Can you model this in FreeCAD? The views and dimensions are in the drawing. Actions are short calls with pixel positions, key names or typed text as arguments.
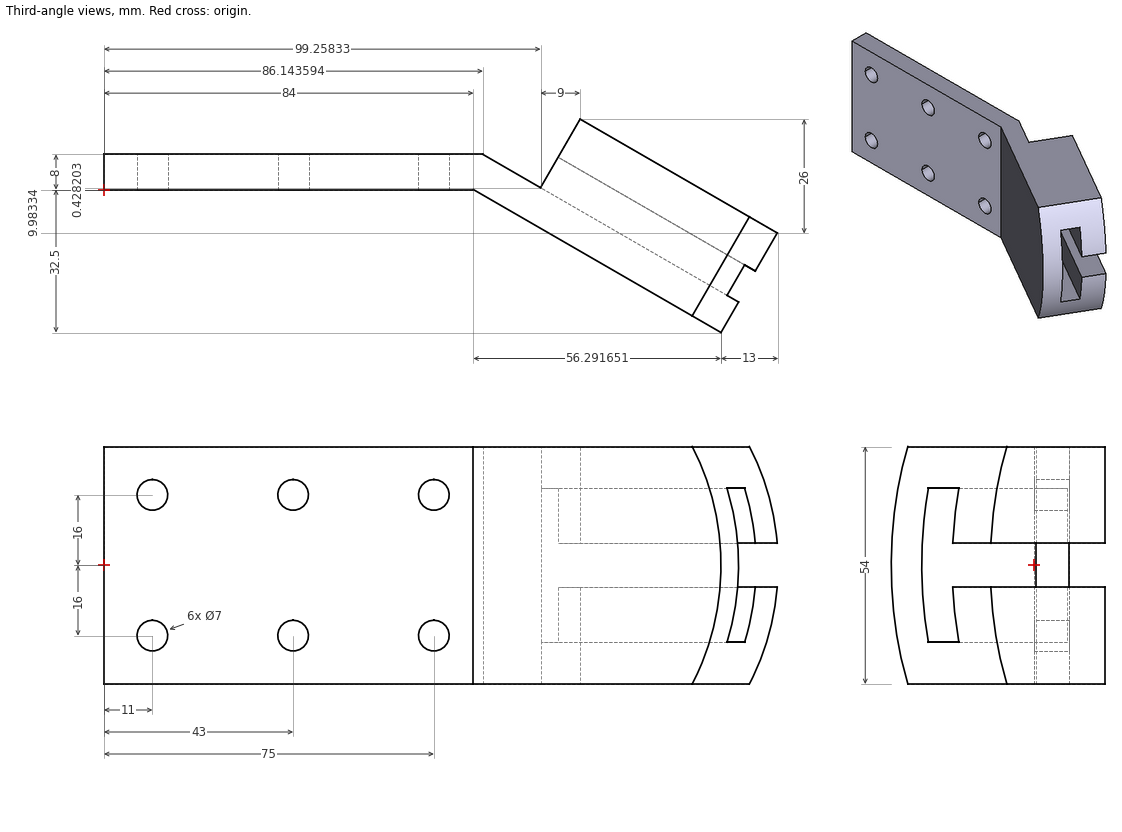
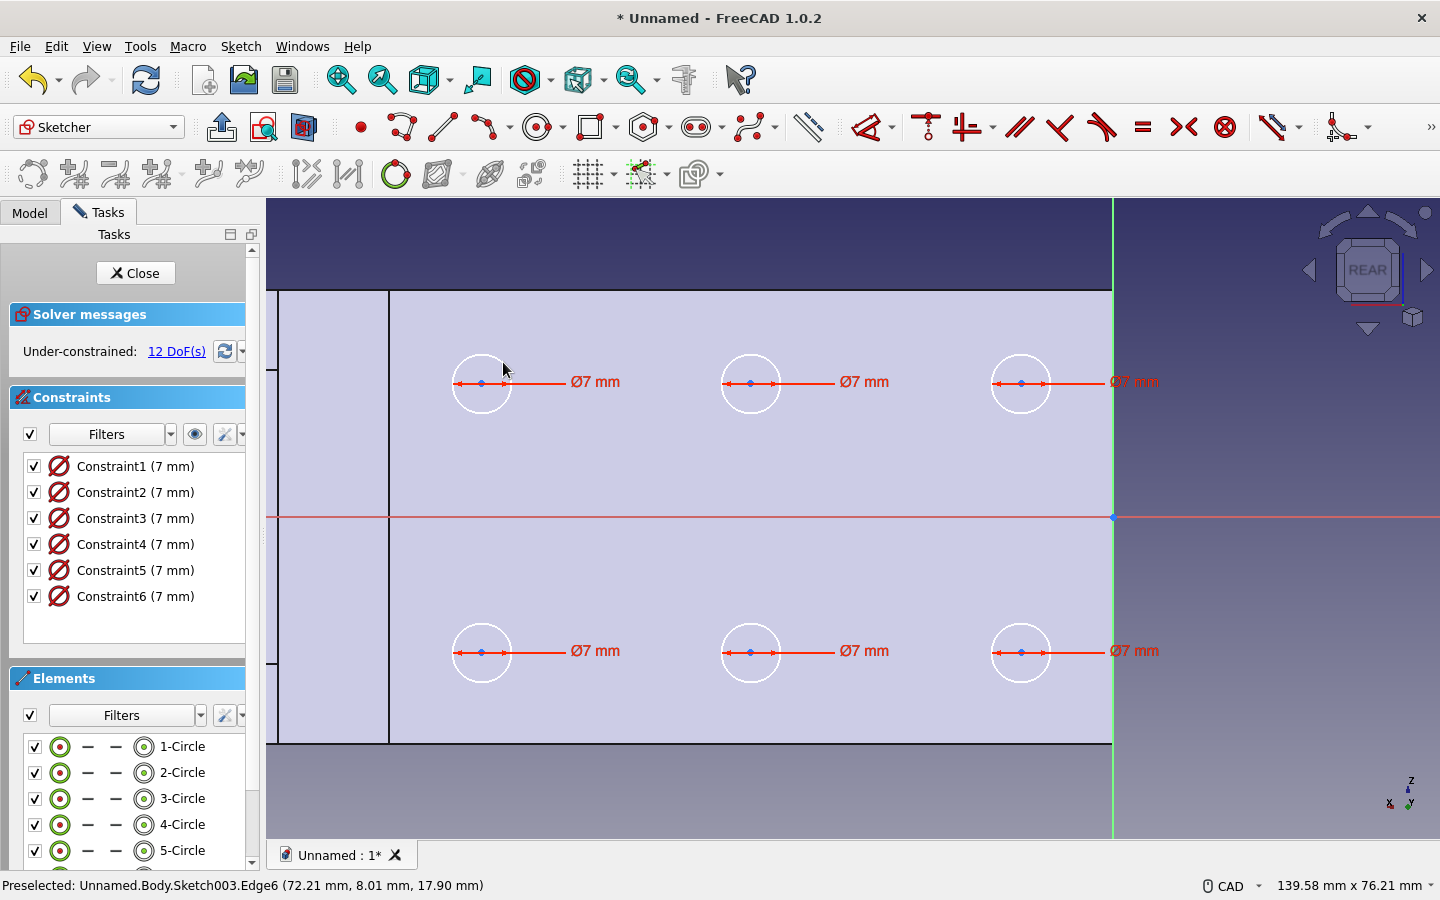
click(1021, 653)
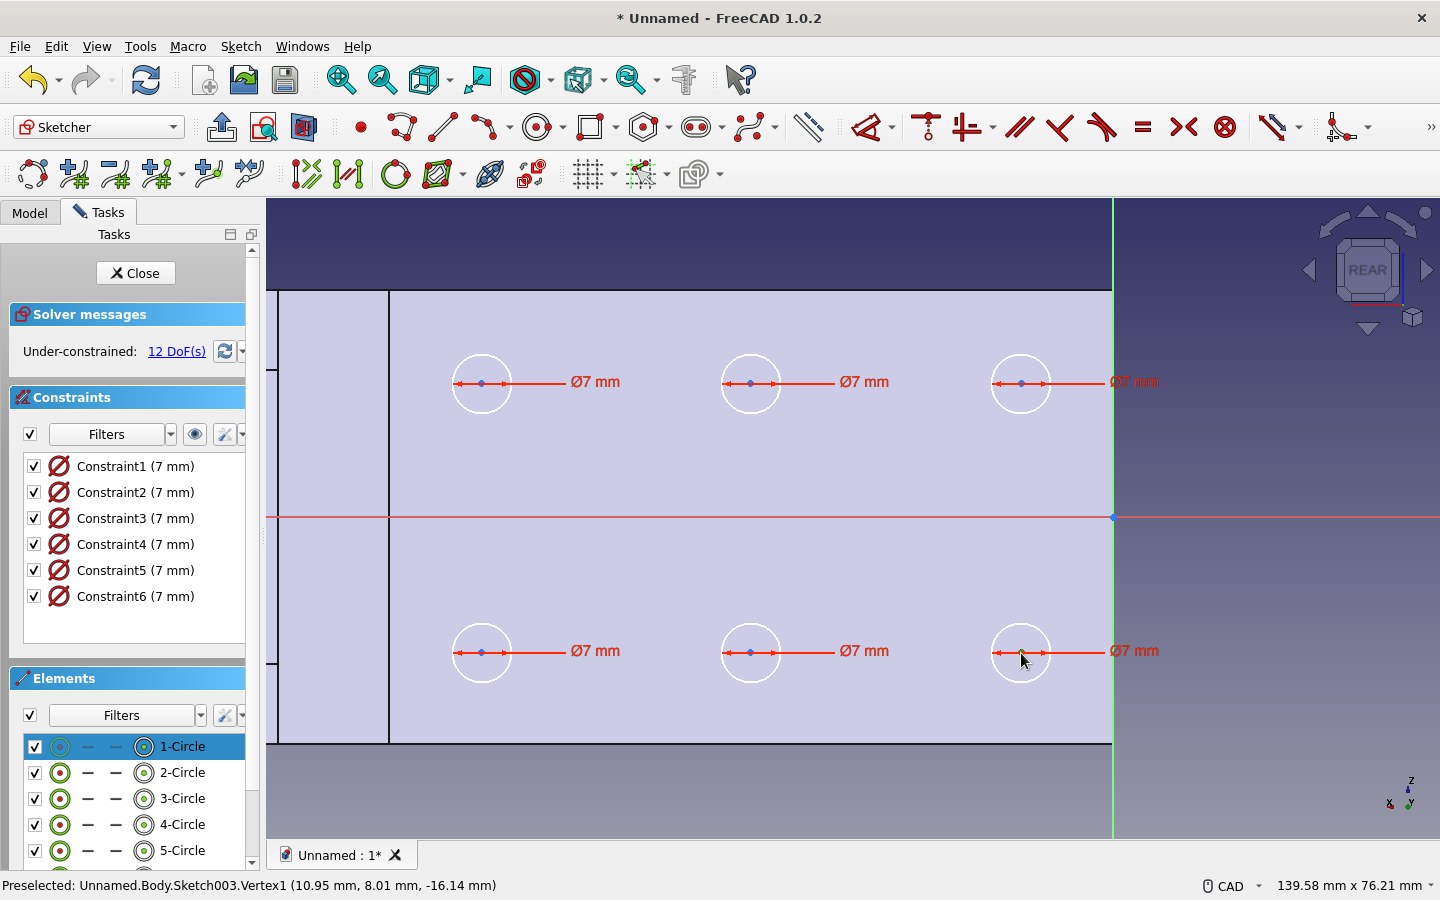
click(751, 653)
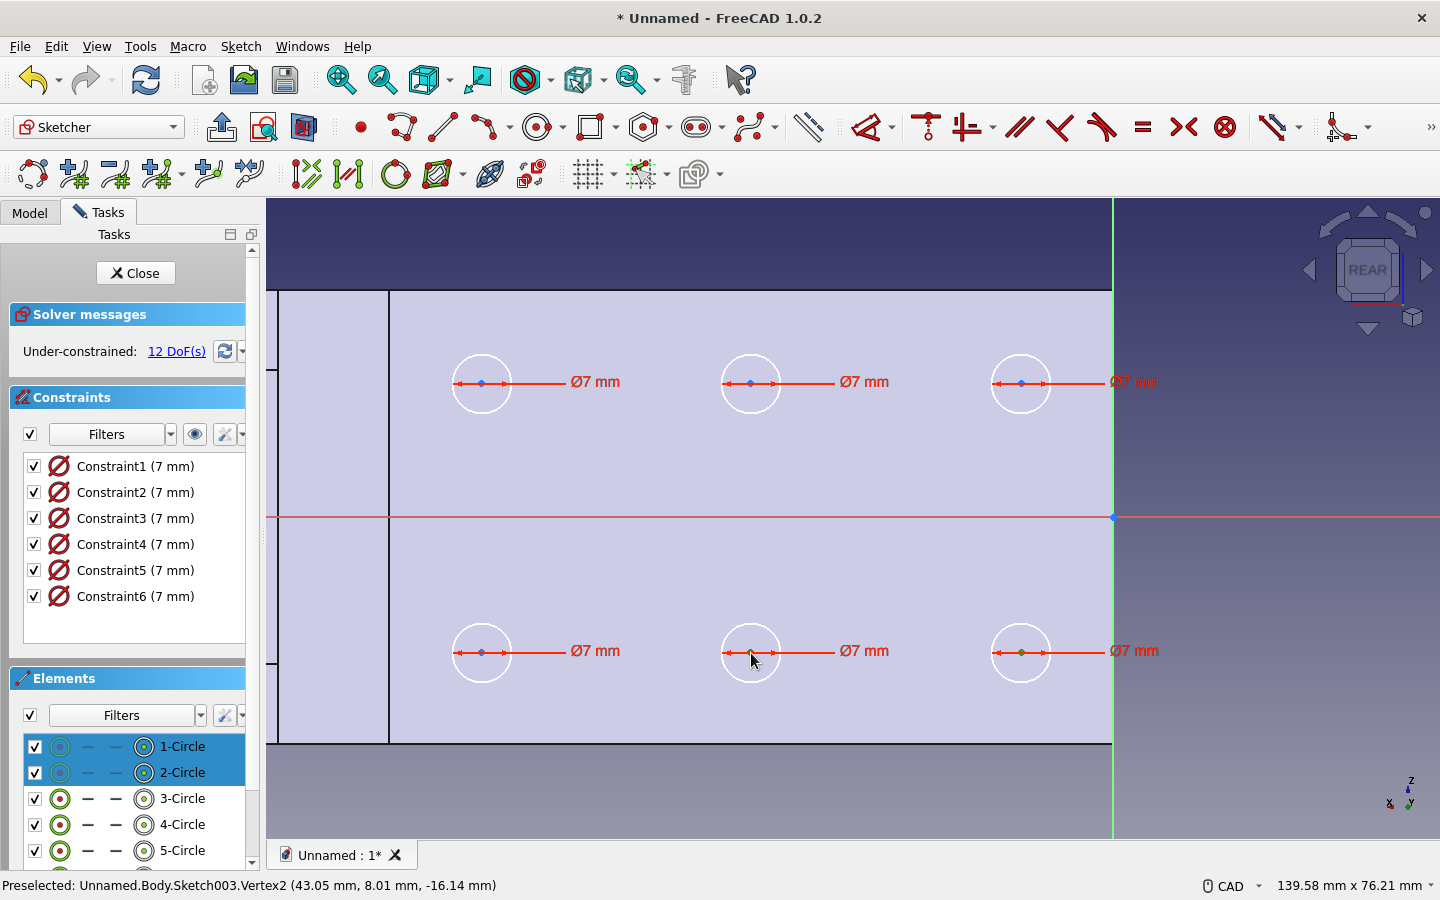
key(h)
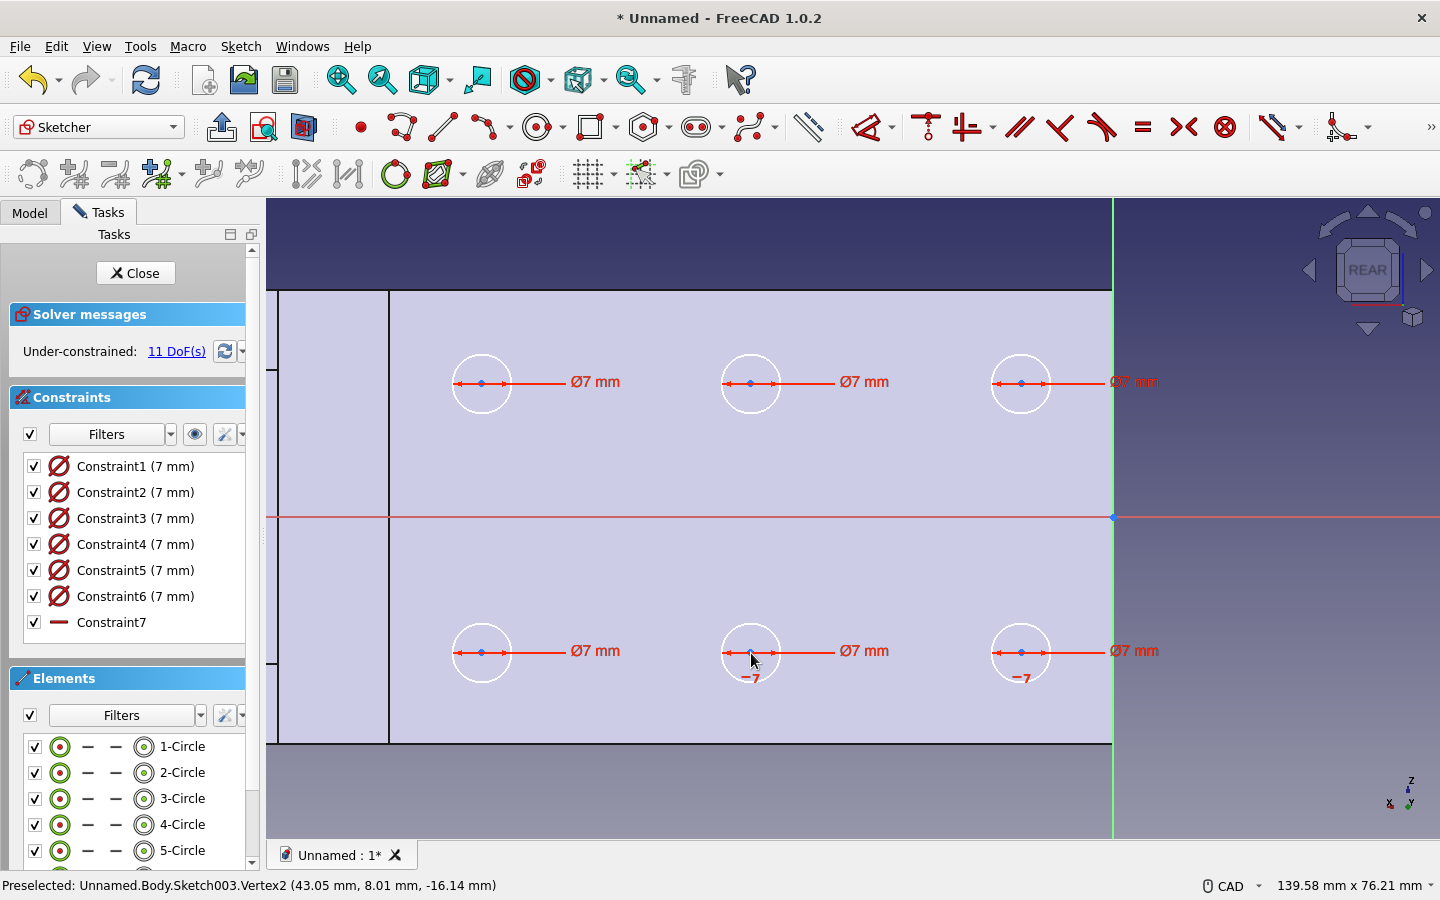
click(751, 653)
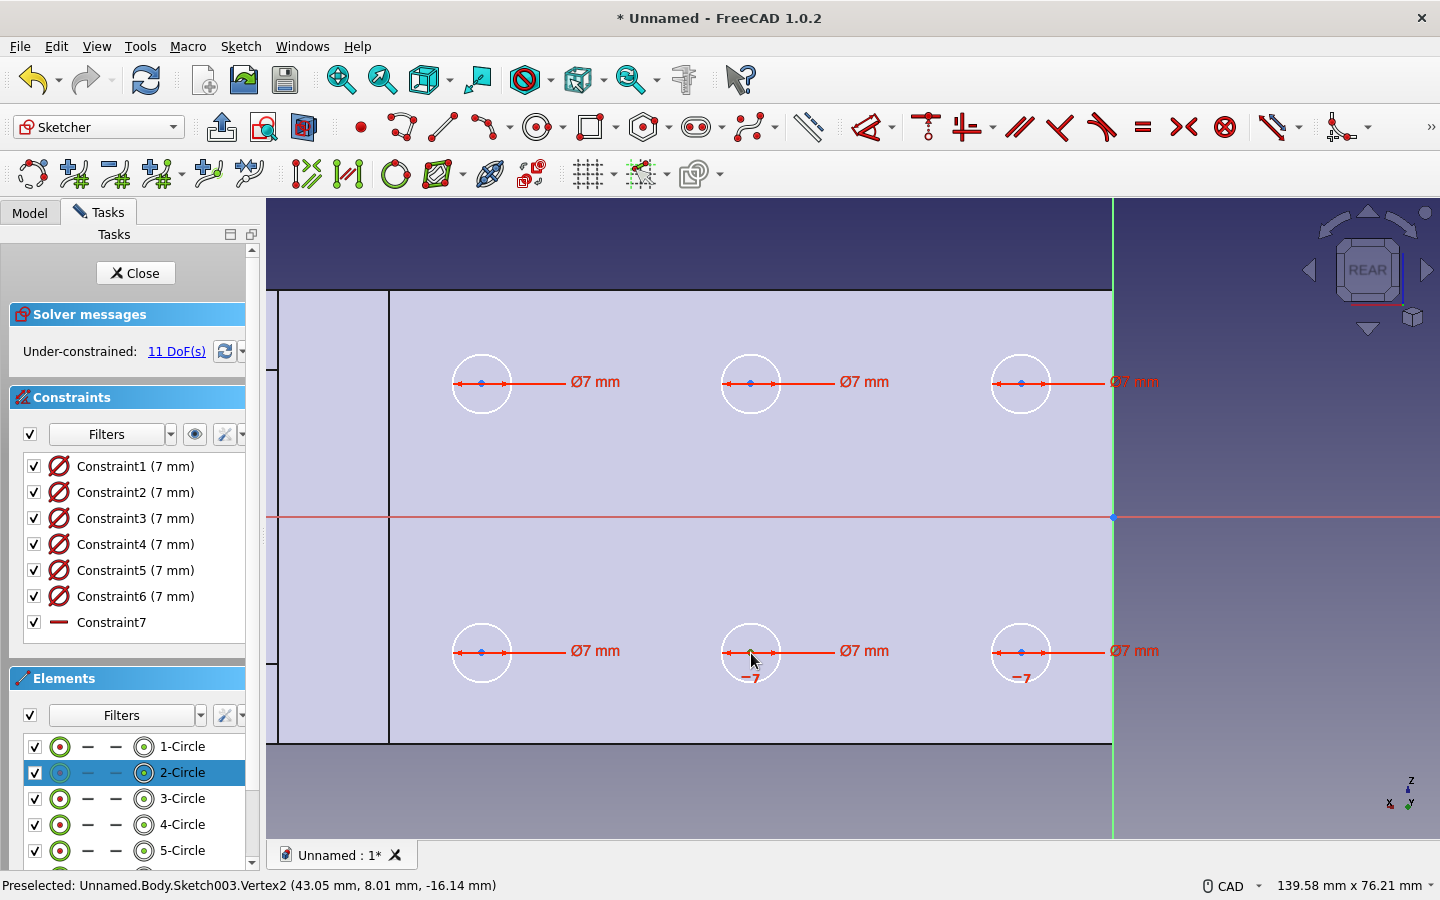
click(482, 653)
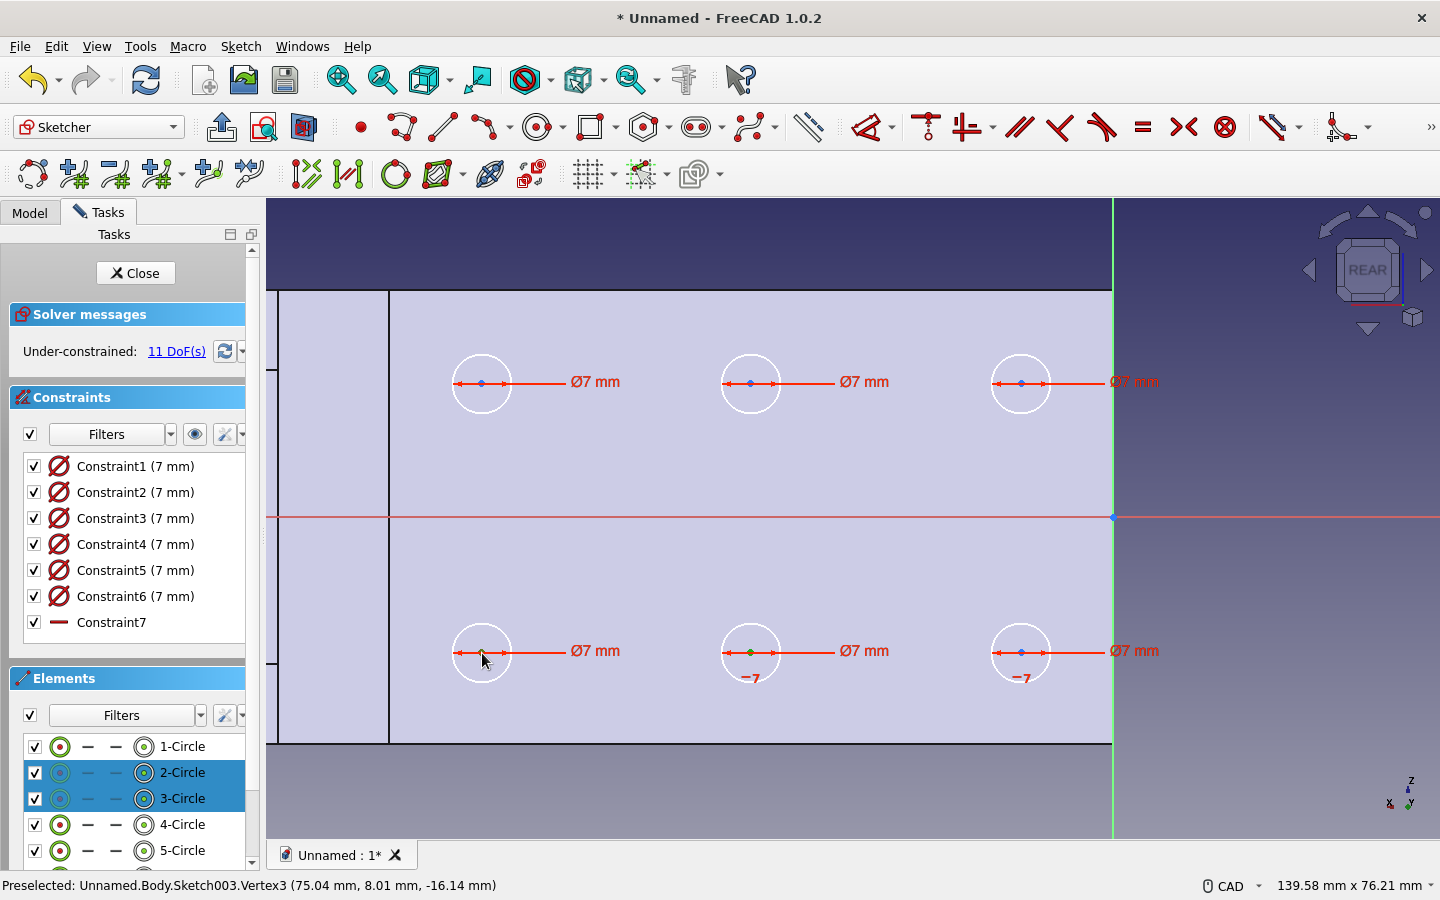
key(h)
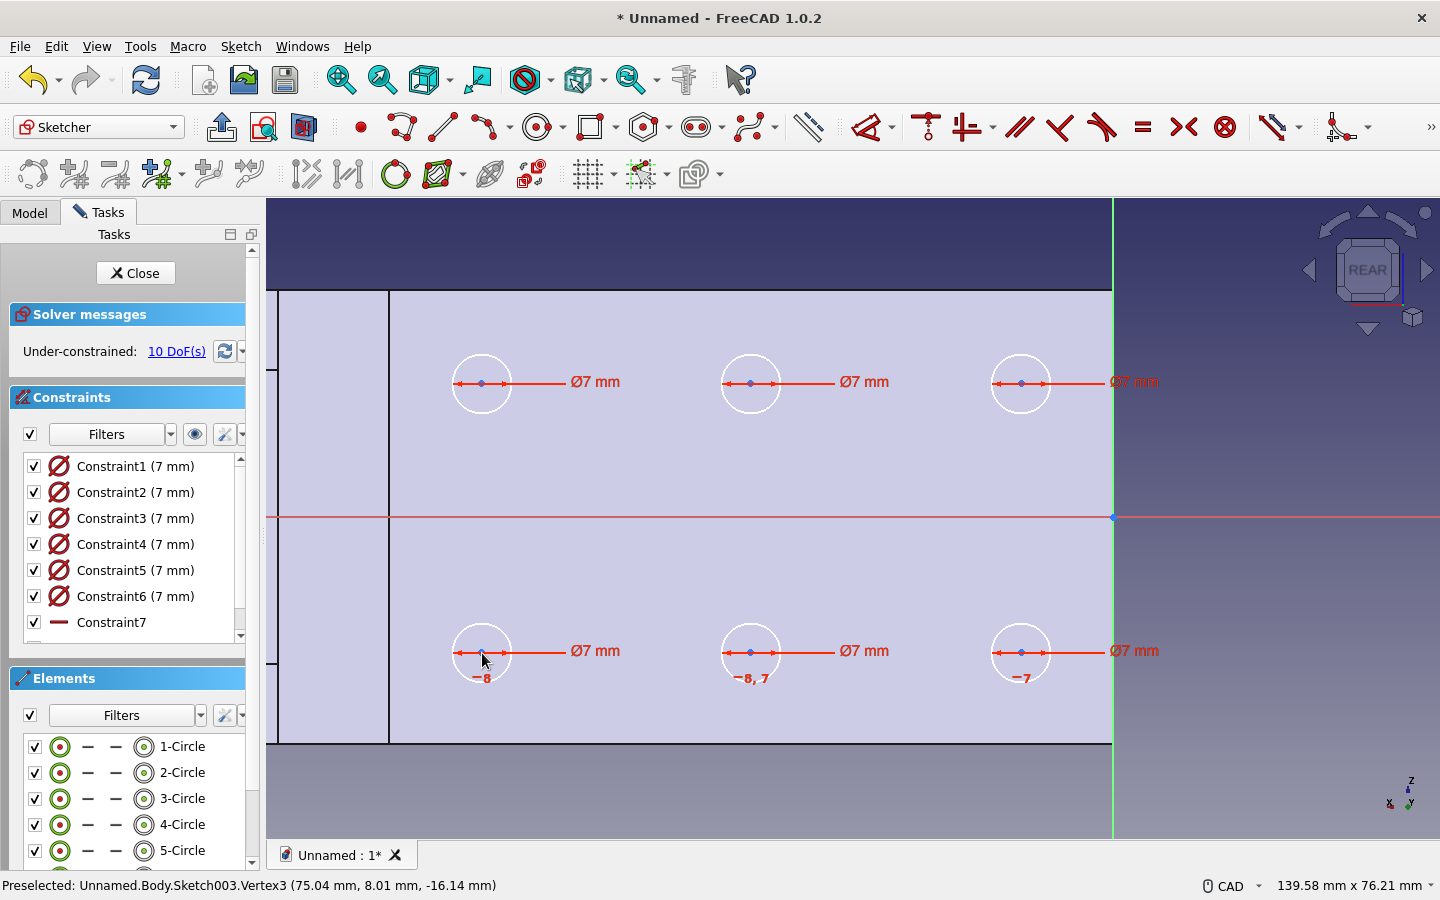
click(1021, 653)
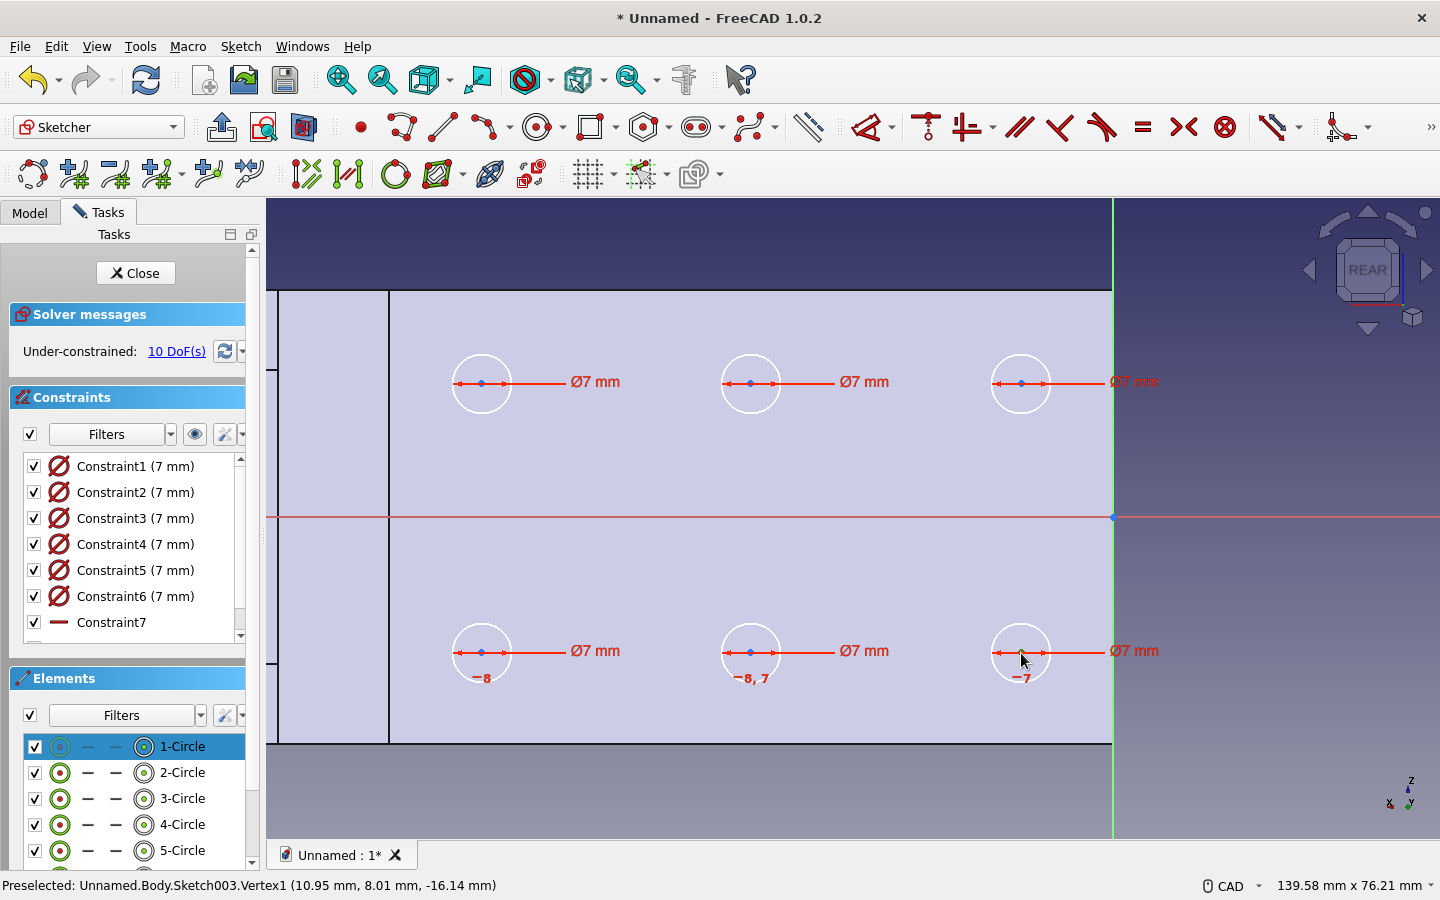
click(1021, 384)